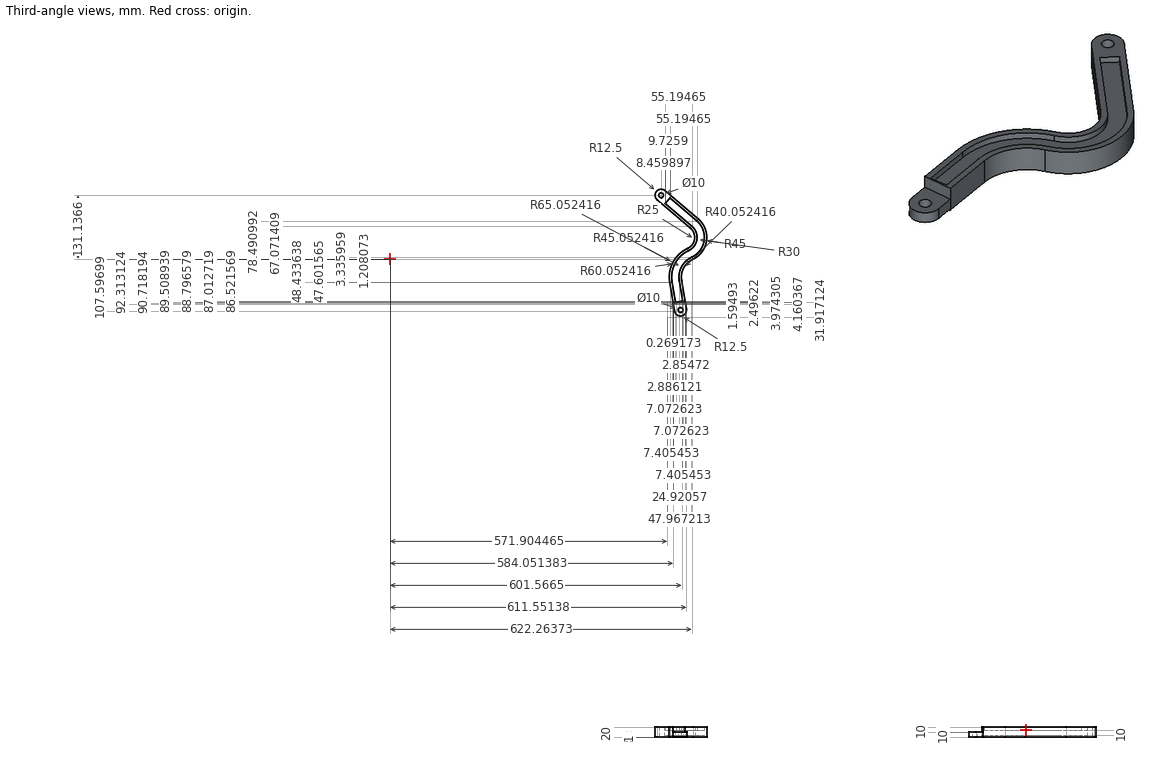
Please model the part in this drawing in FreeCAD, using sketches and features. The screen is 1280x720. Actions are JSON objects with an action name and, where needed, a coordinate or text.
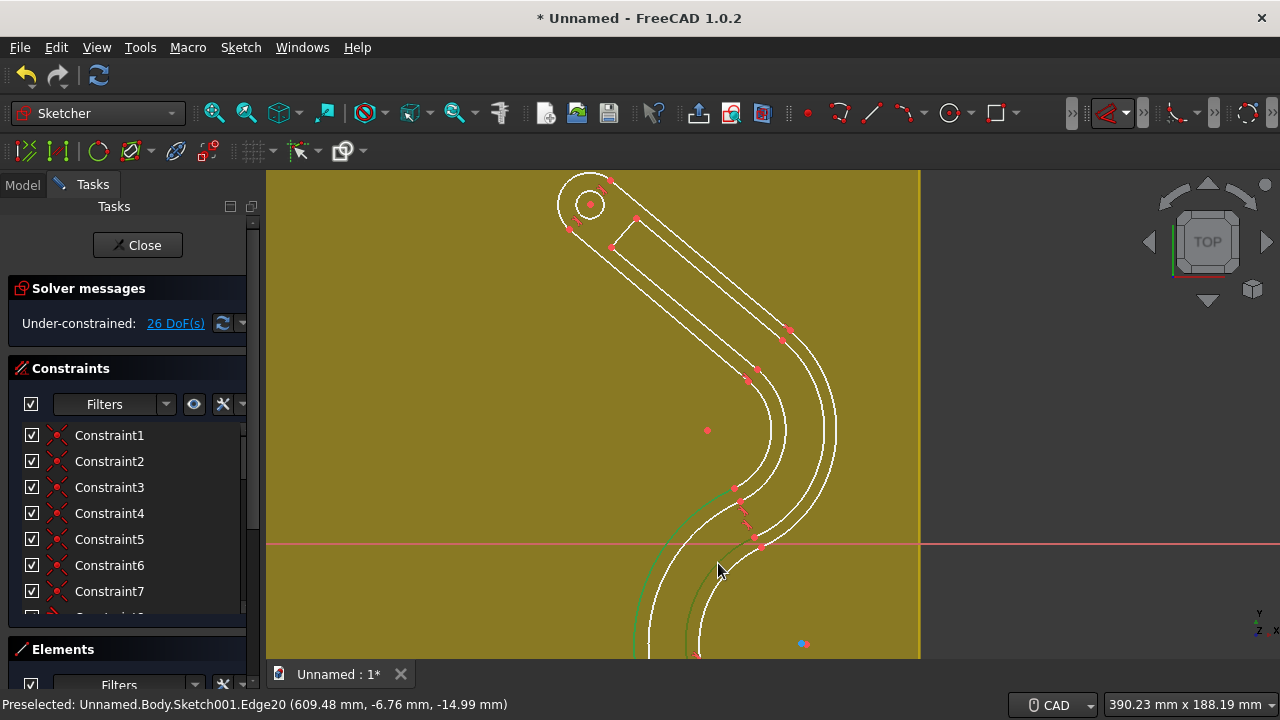
{"action": "key", "text": "c"}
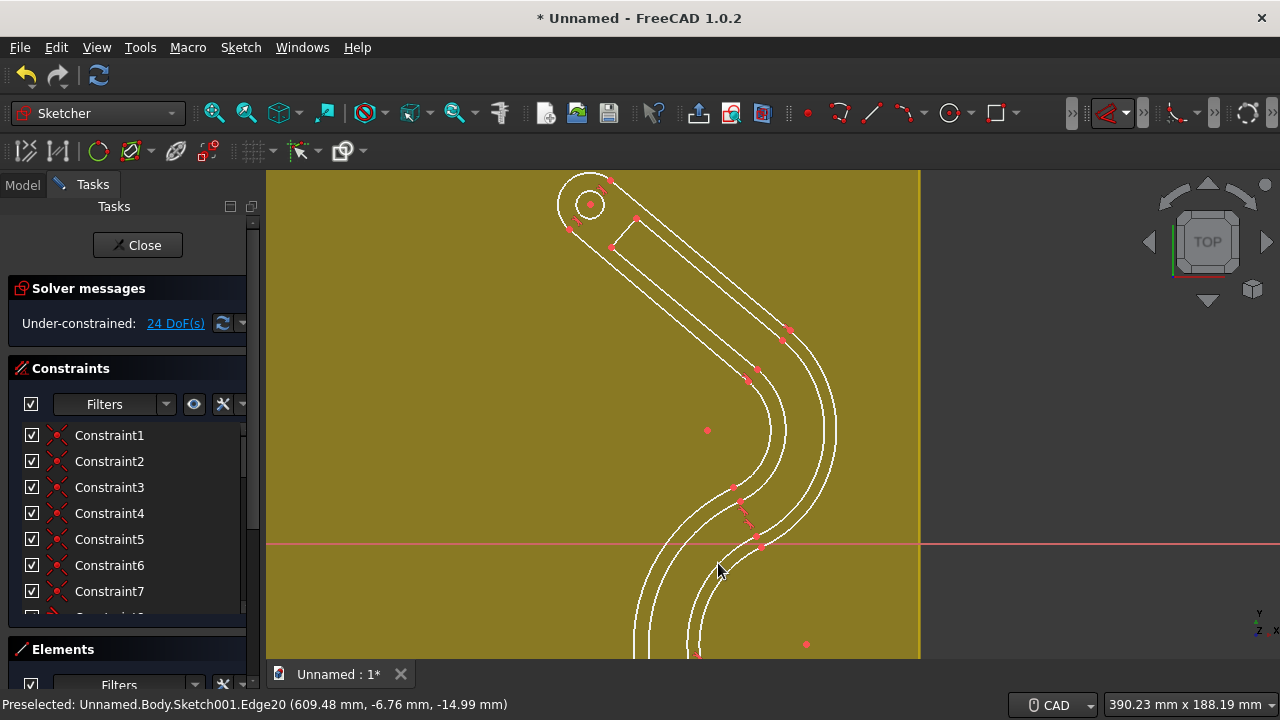
{"action": "scroll", "coordinate": [558, 203], "scroll_direction": "up", "scroll_amount": 2}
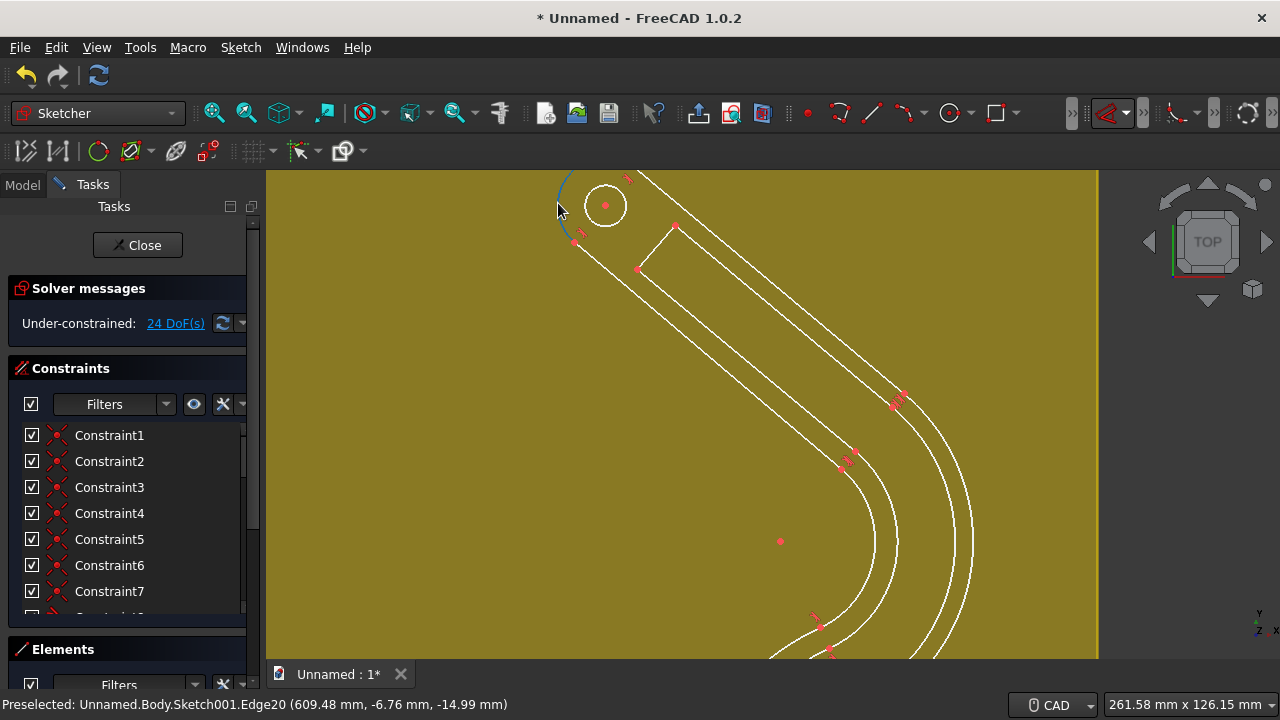
{"action": "left_click", "coordinate": [558, 202]}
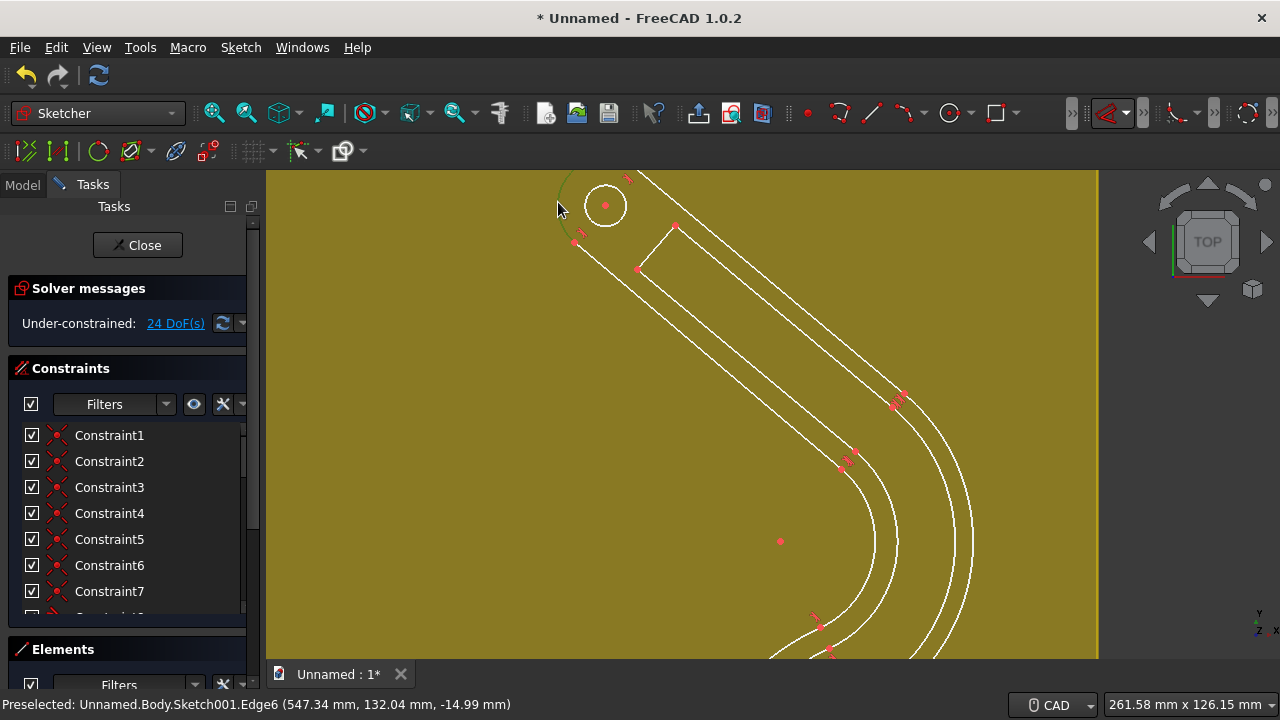
{"action": "left_click", "coordinate": [1128, 114]}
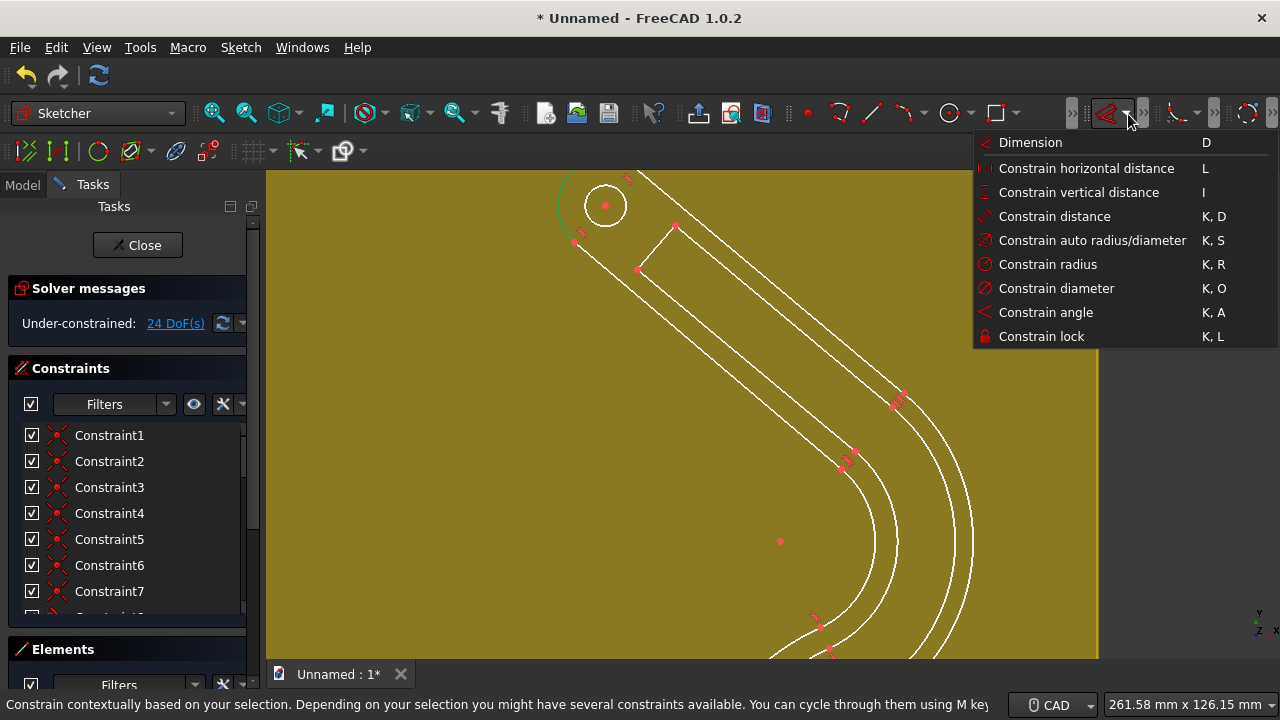
{"action": "left_click", "coordinate": [1126, 264]}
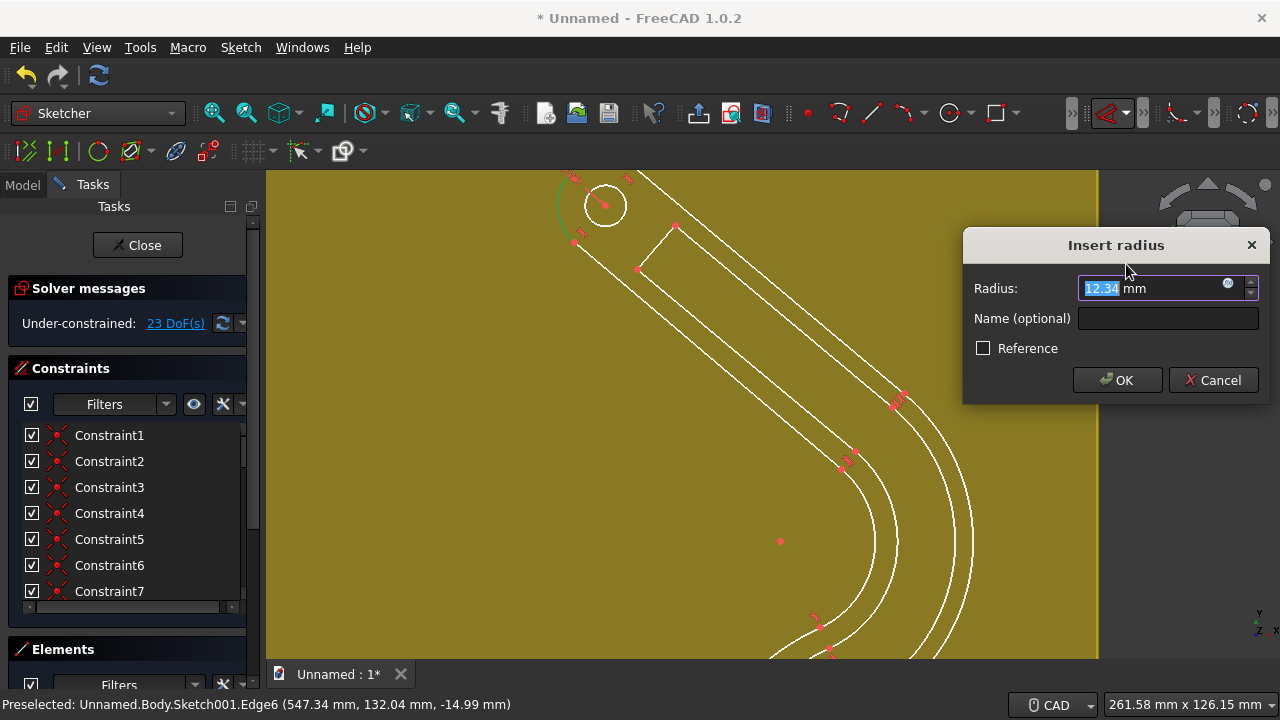
{"action": "type", "text": "12.5"}
{"action": "key", "text": "Return"}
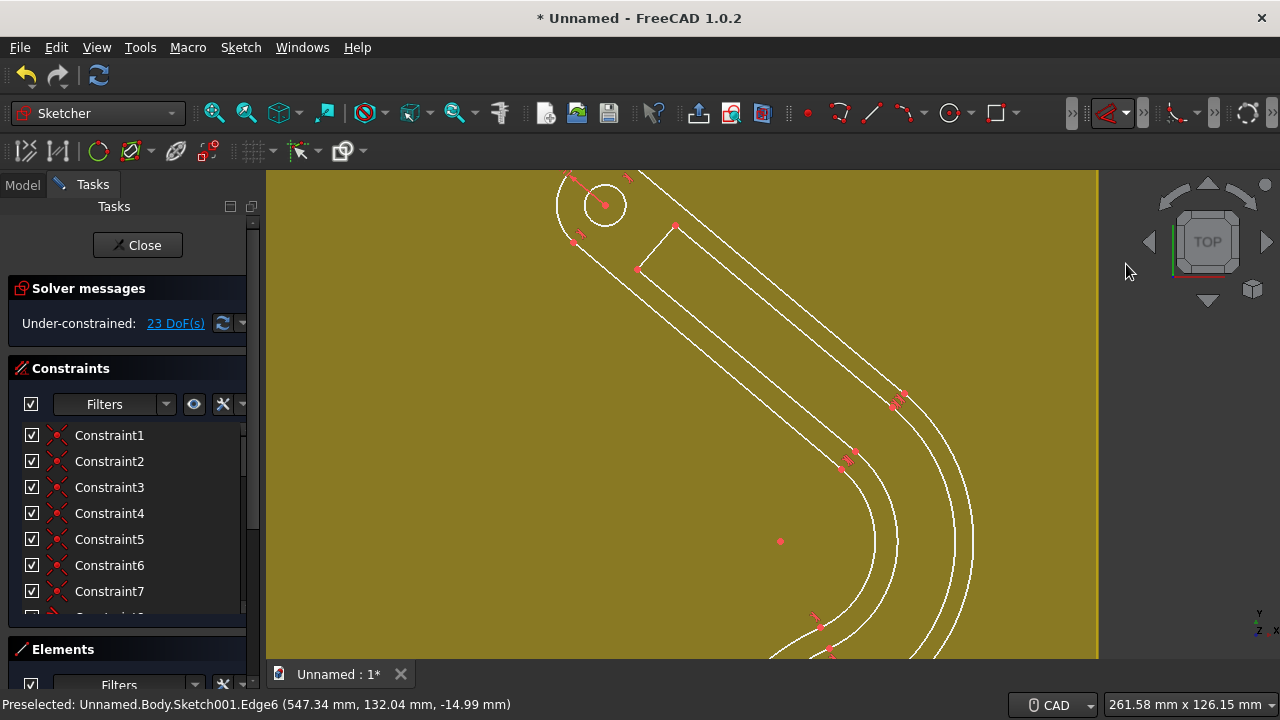
{"action": "left_click", "coordinate": [862, 590]}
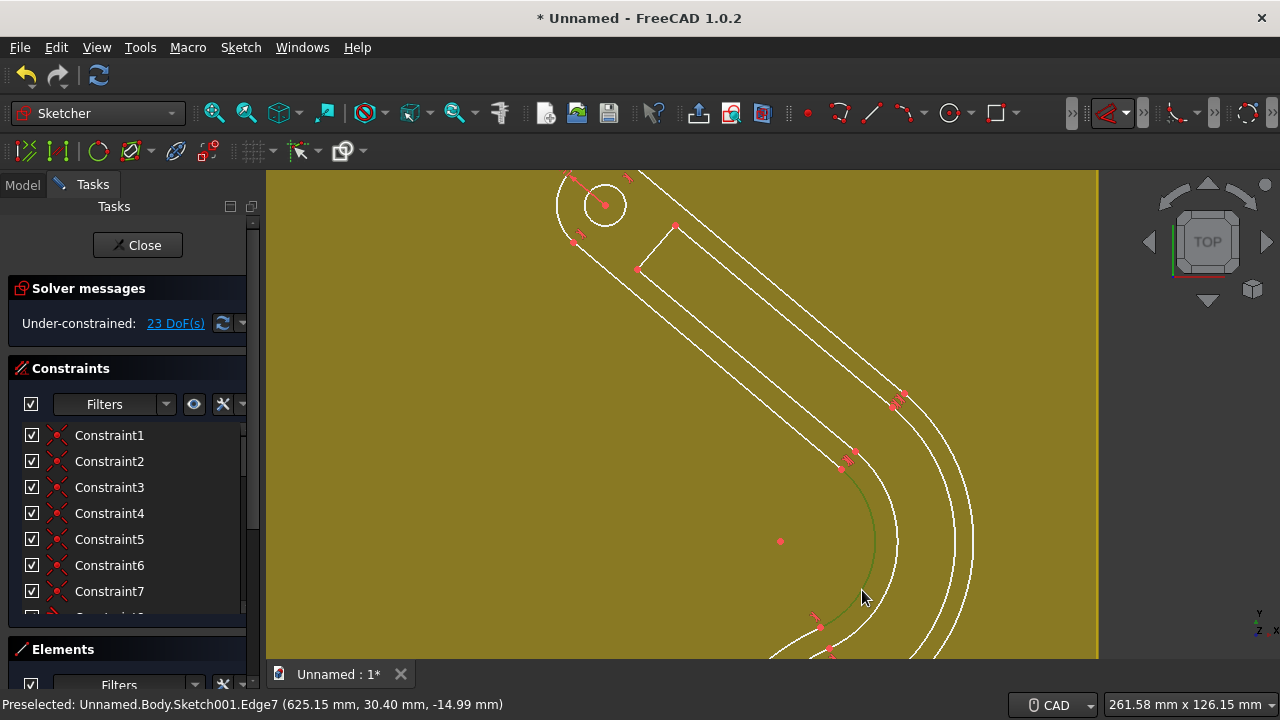
{"action": "key", "text": "k r"}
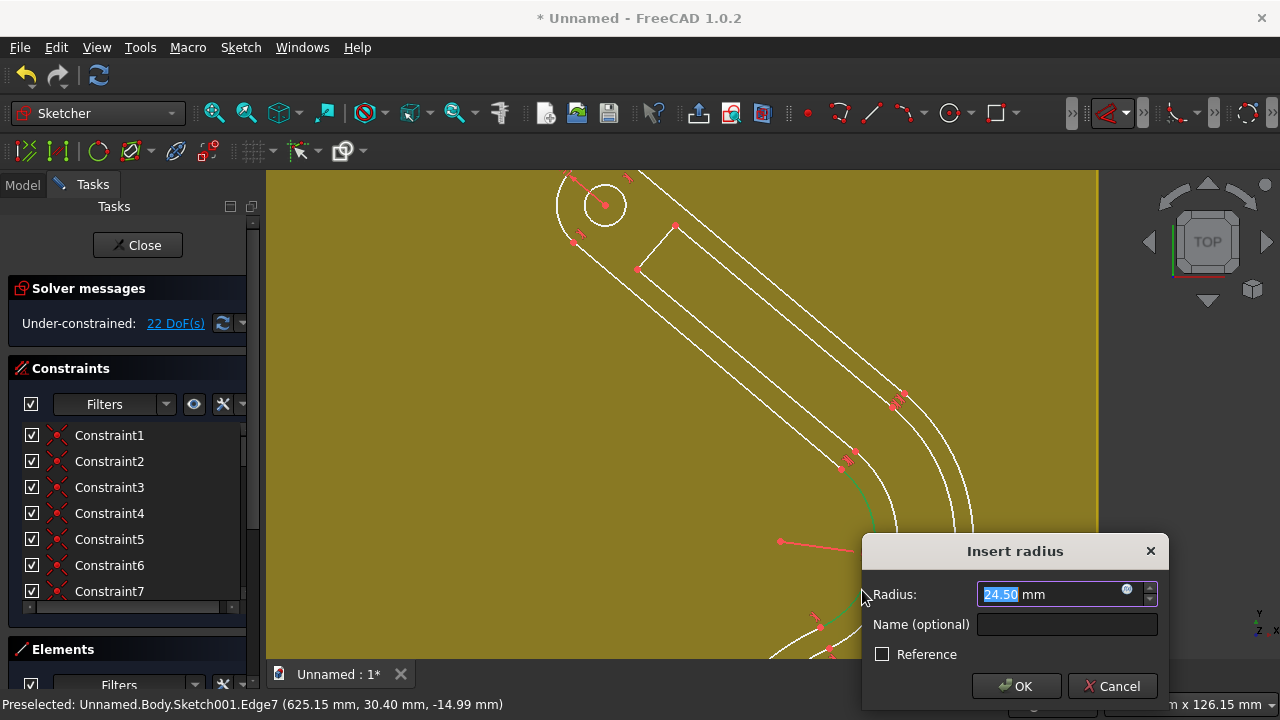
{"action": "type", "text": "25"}
{"action": "key", "text": "Return"}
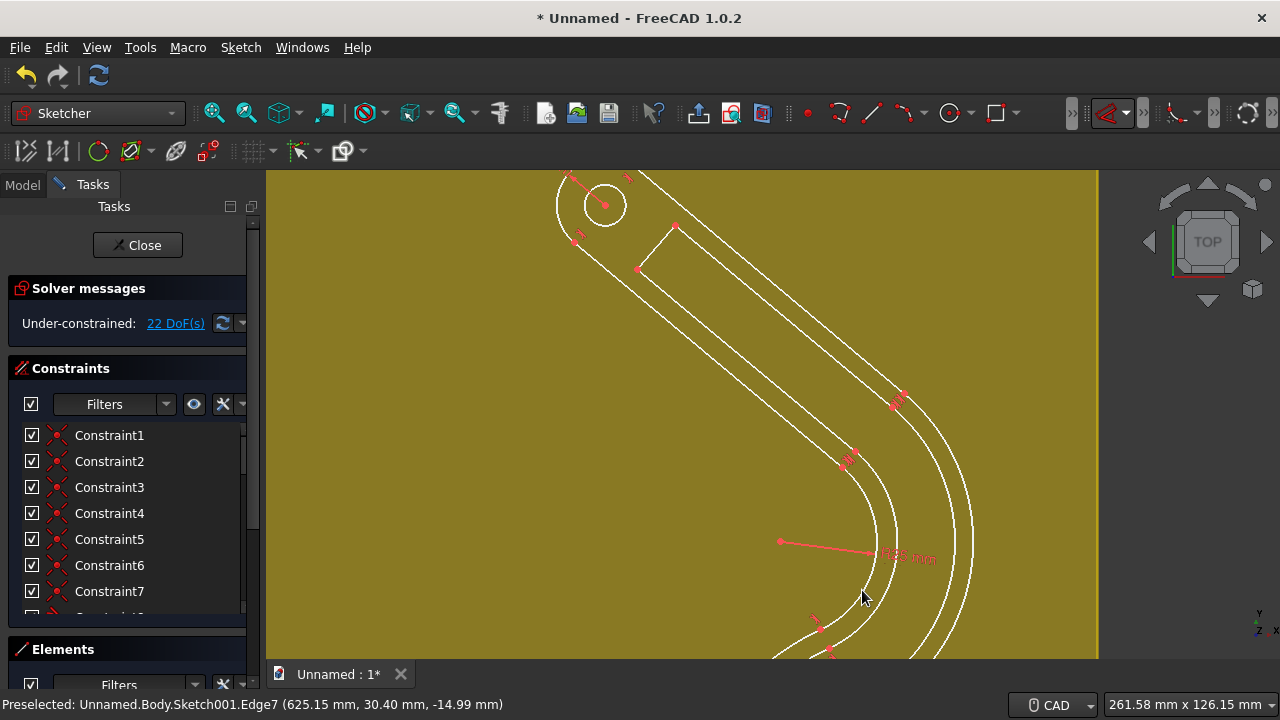
{"action": "scroll", "coordinate": [668, 296], "scroll_direction": "down", "scroll_amount": 5}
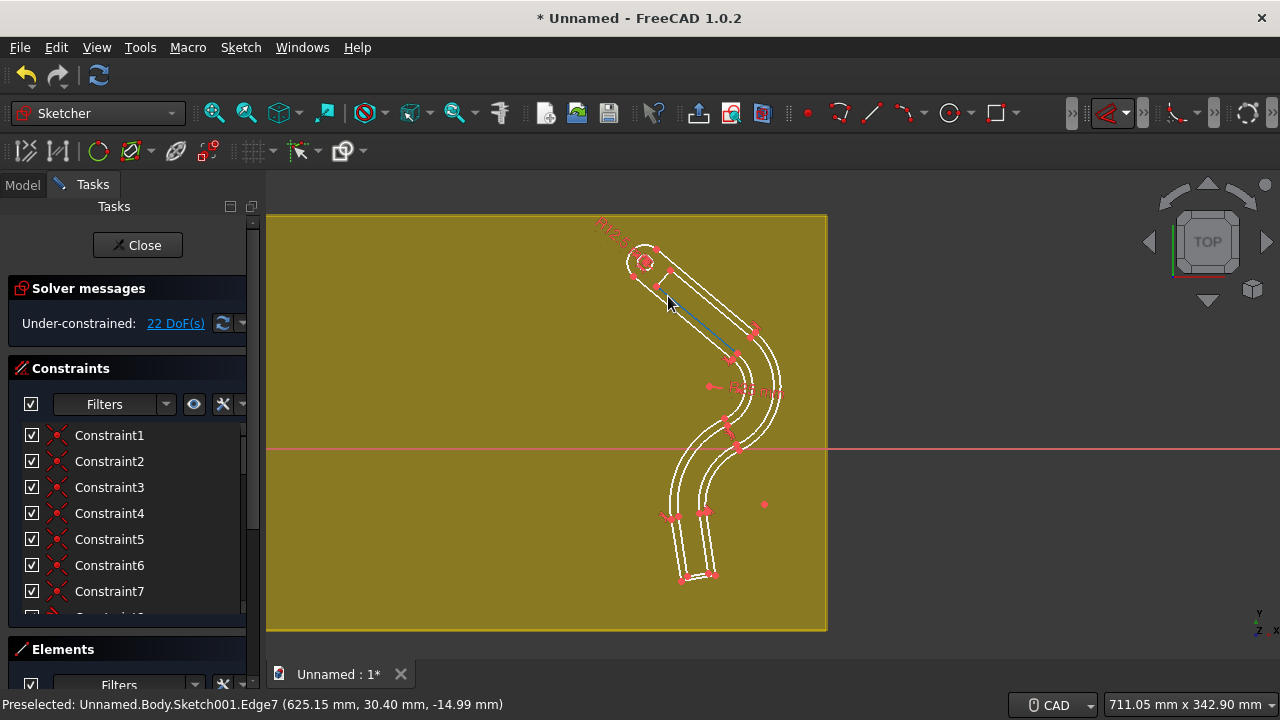
{"action": "scroll", "coordinate": [695, 440], "scroll_direction": "up", "scroll_amount": 4}